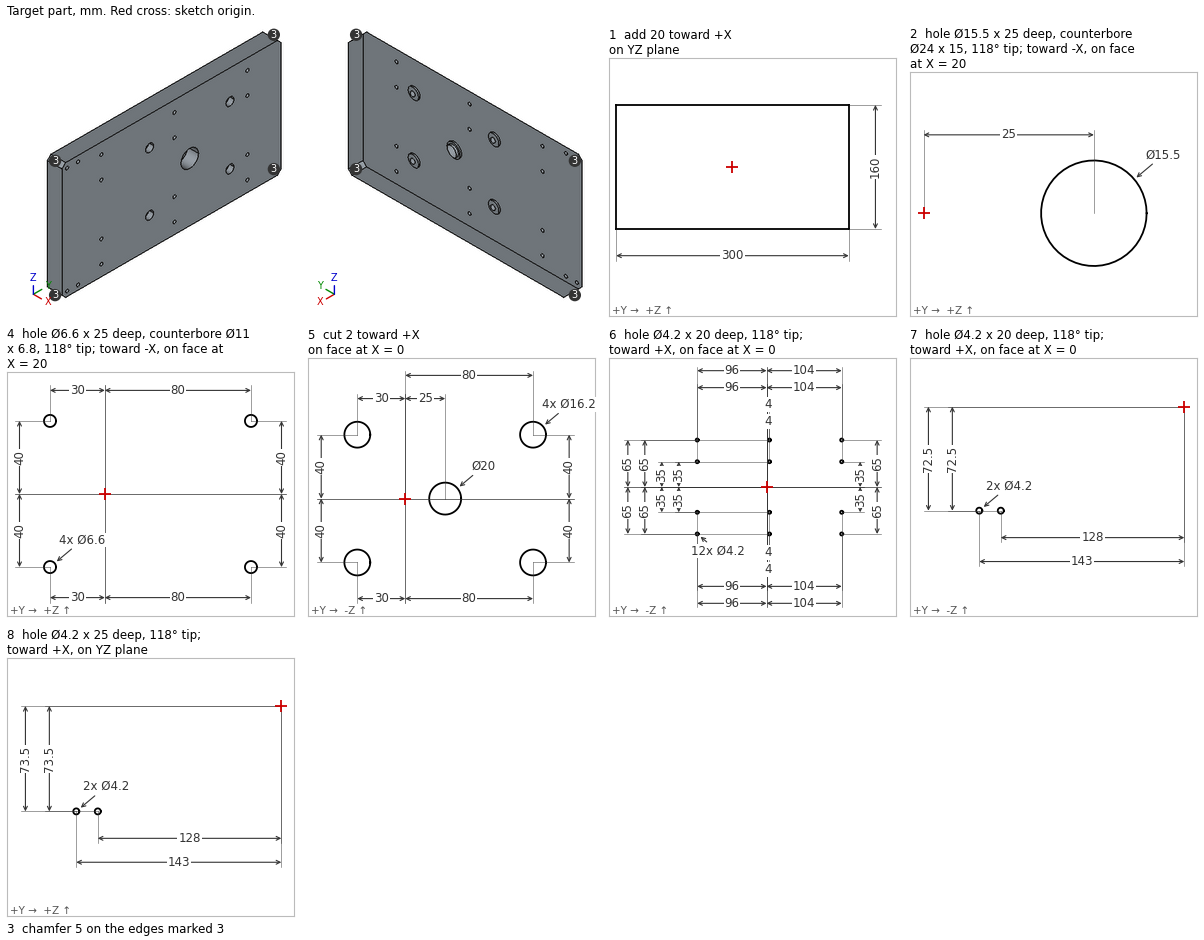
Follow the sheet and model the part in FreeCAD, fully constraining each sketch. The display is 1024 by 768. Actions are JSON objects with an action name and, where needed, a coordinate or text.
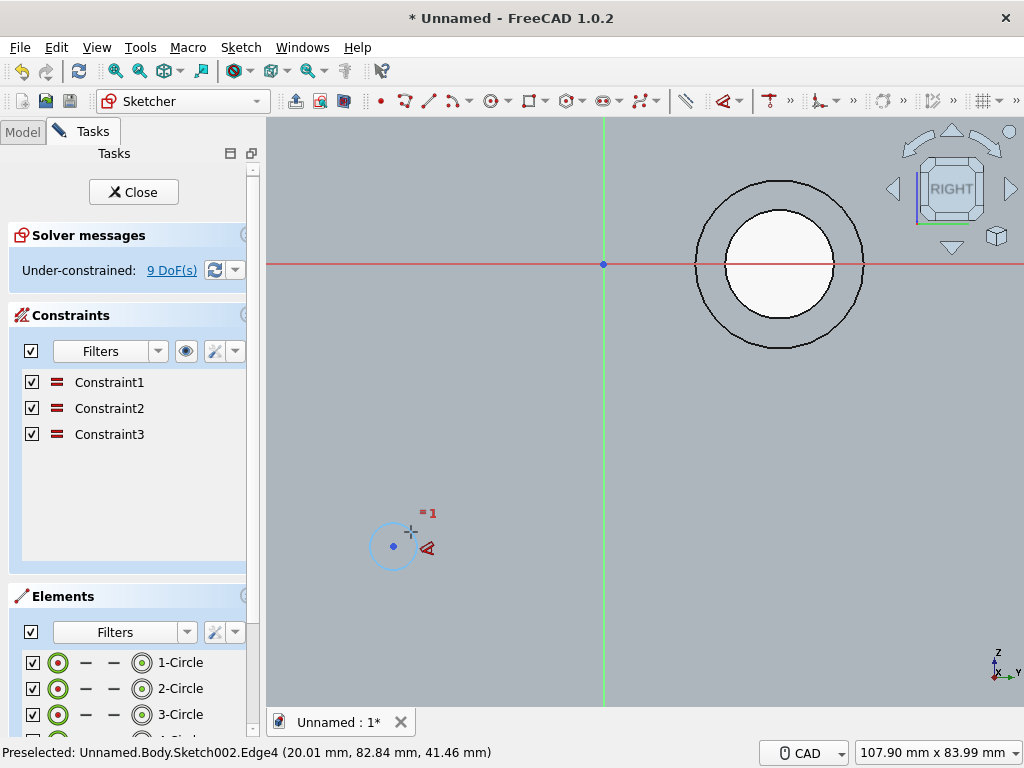
{"action": "left_click", "coordinate": [410, 530]}
{"action": "left_click", "coordinate": [433, 507]}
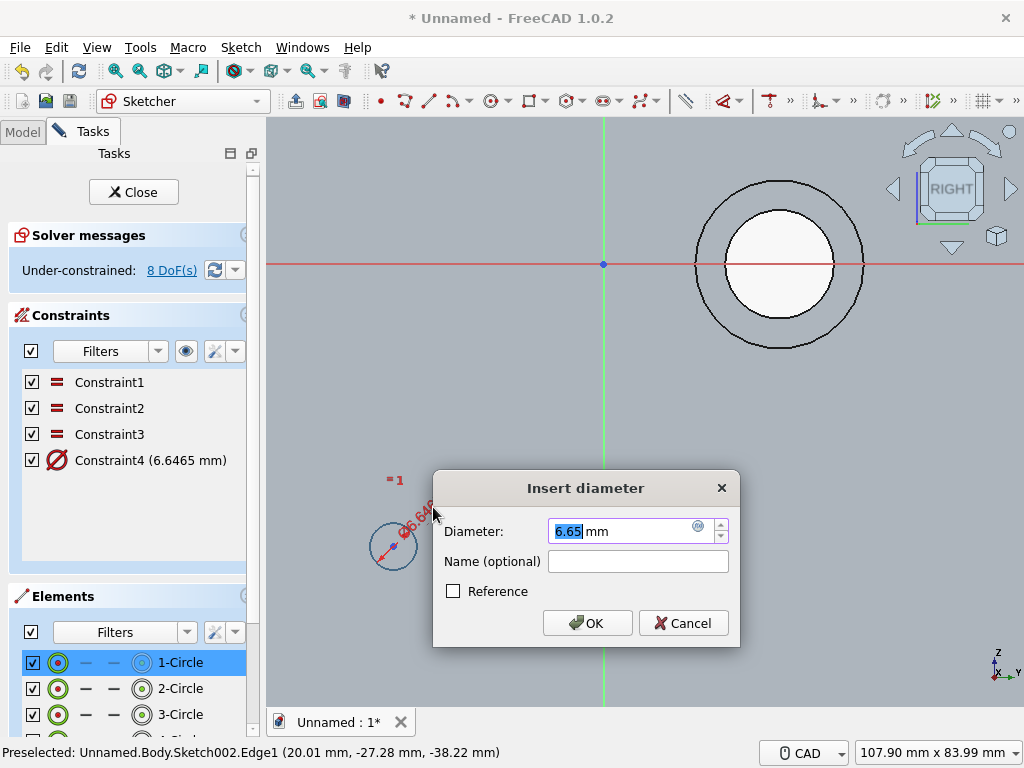
{"action": "type", "text": "6.6"}
{"action": "key", "text": "Return"}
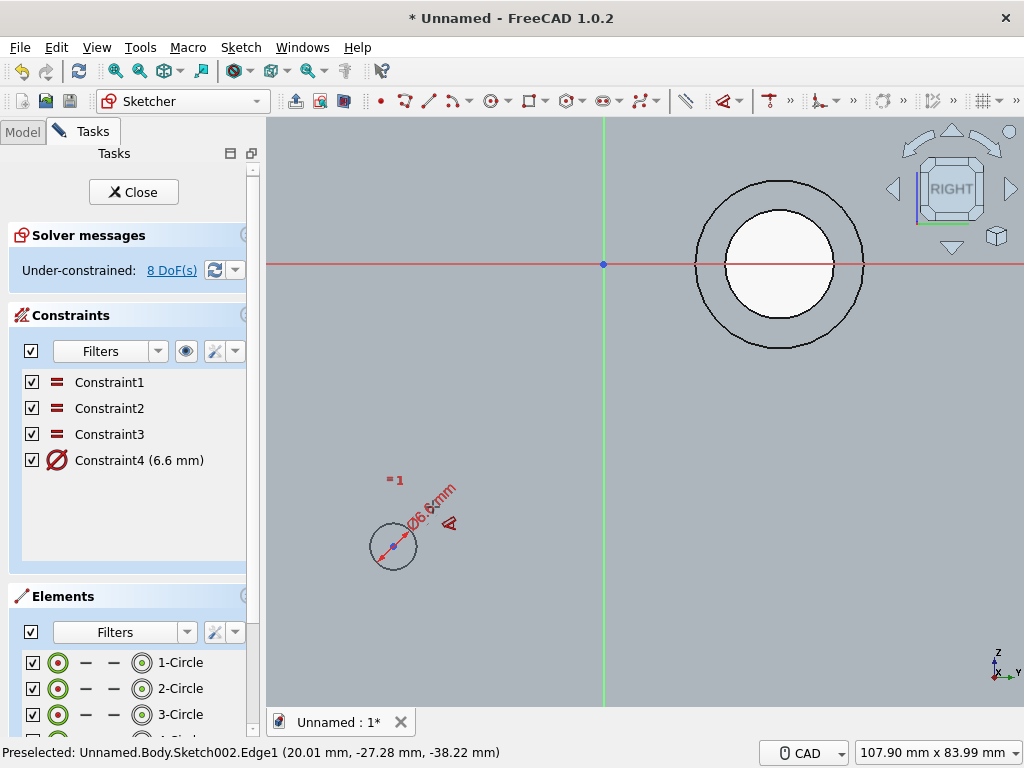
{"action": "left_click", "coordinate": [393, 547]}
{"action": "left_click", "coordinate": [499, 581]}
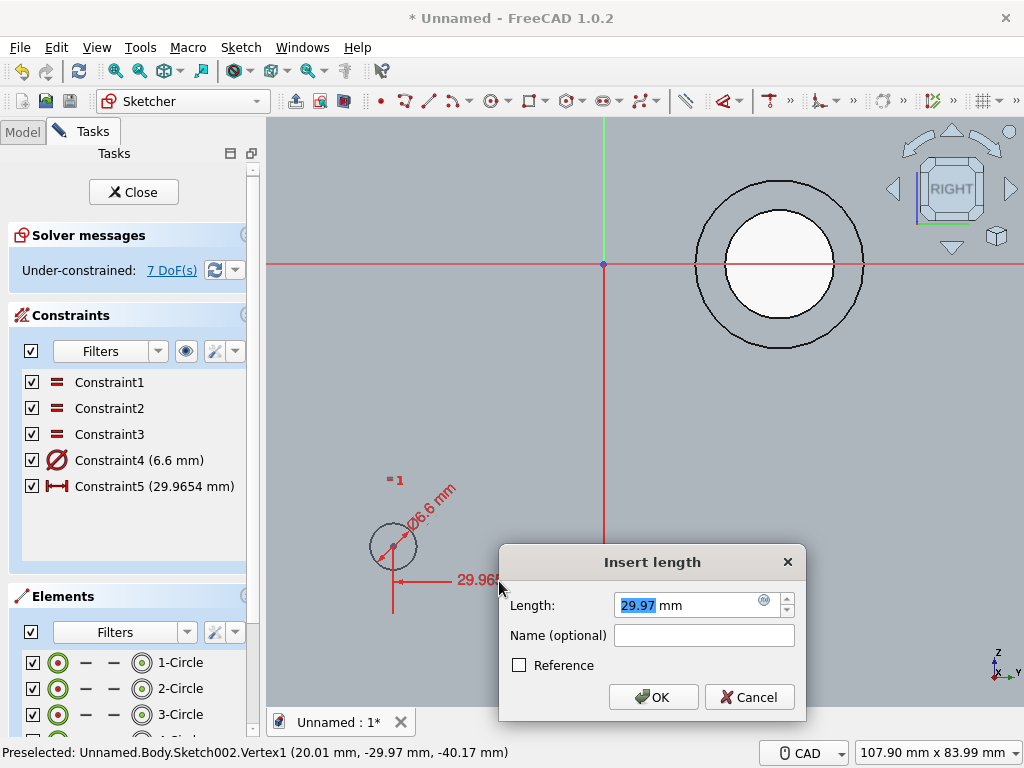
{"action": "type", "text": "30"}
{"action": "key", "text": "Return"}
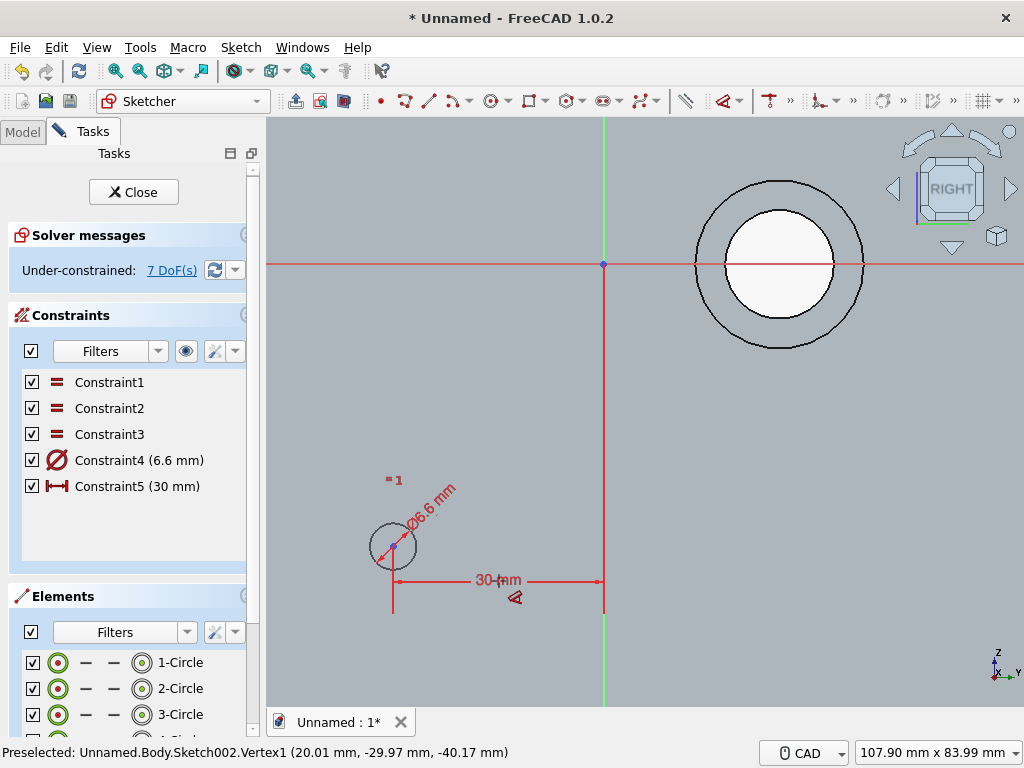
{"action": "left_click", "coordinate": [393, 547]}
{"action": "left_click", "coordinate": [359, 405]}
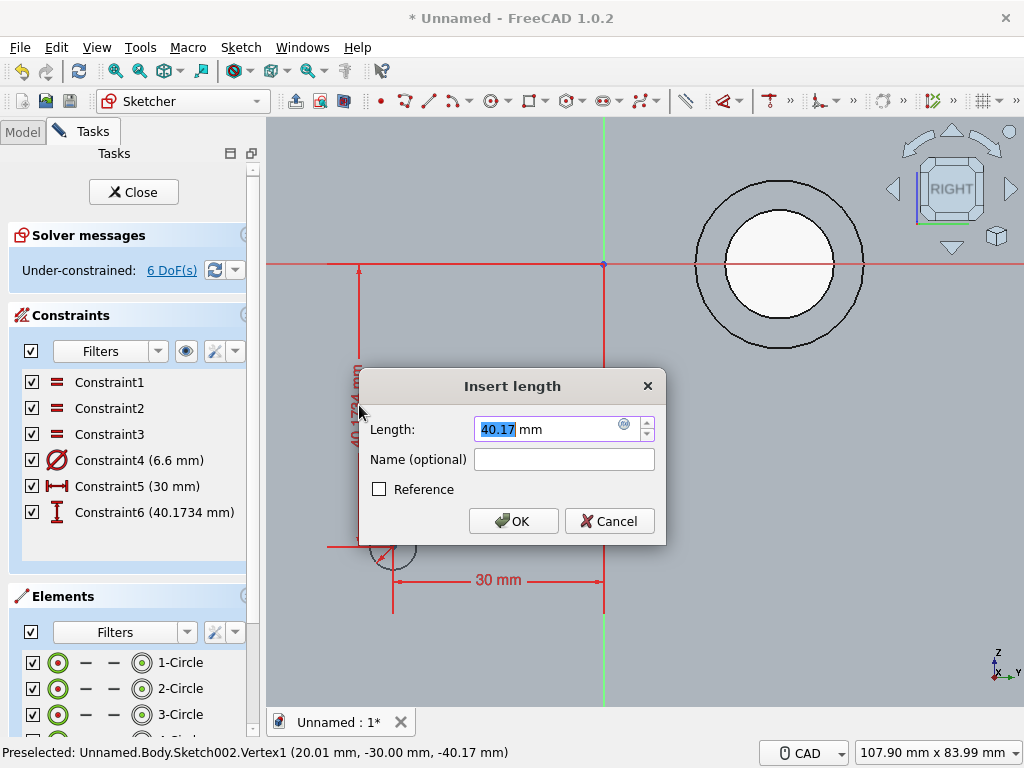
{"action": "type", "text": "40"}
{"action": "key", "text": "Return"}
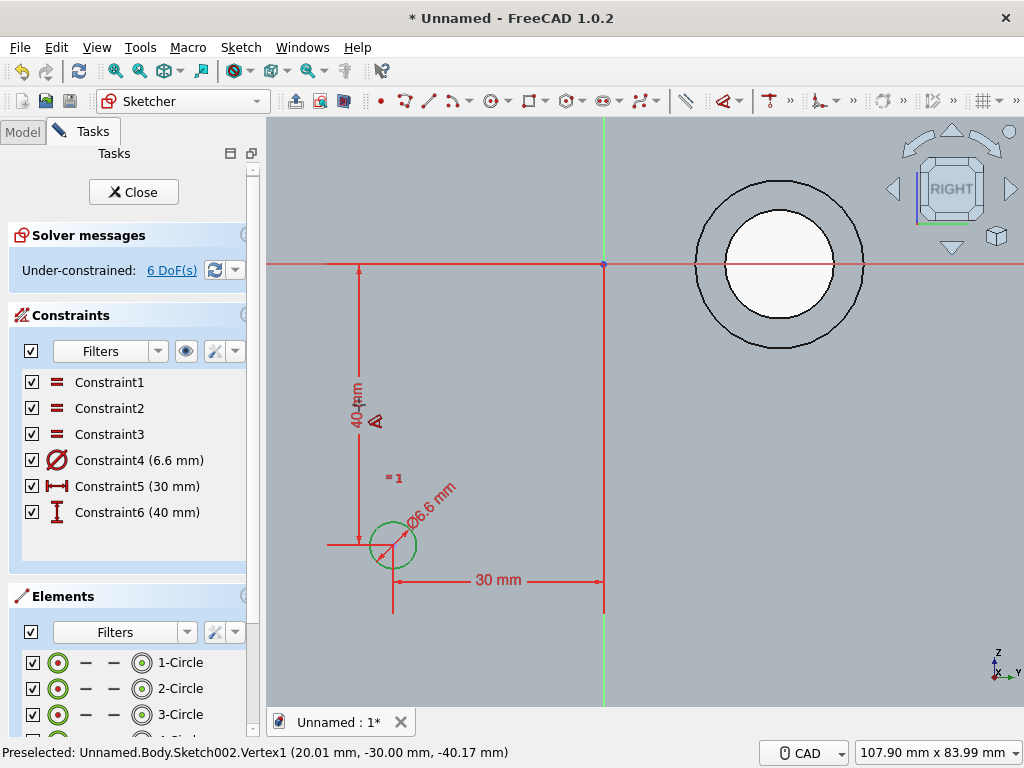
{"action": "scroll", "coordinate": [411, 532], "scroll_direction": "down", "scroll_amount": 4}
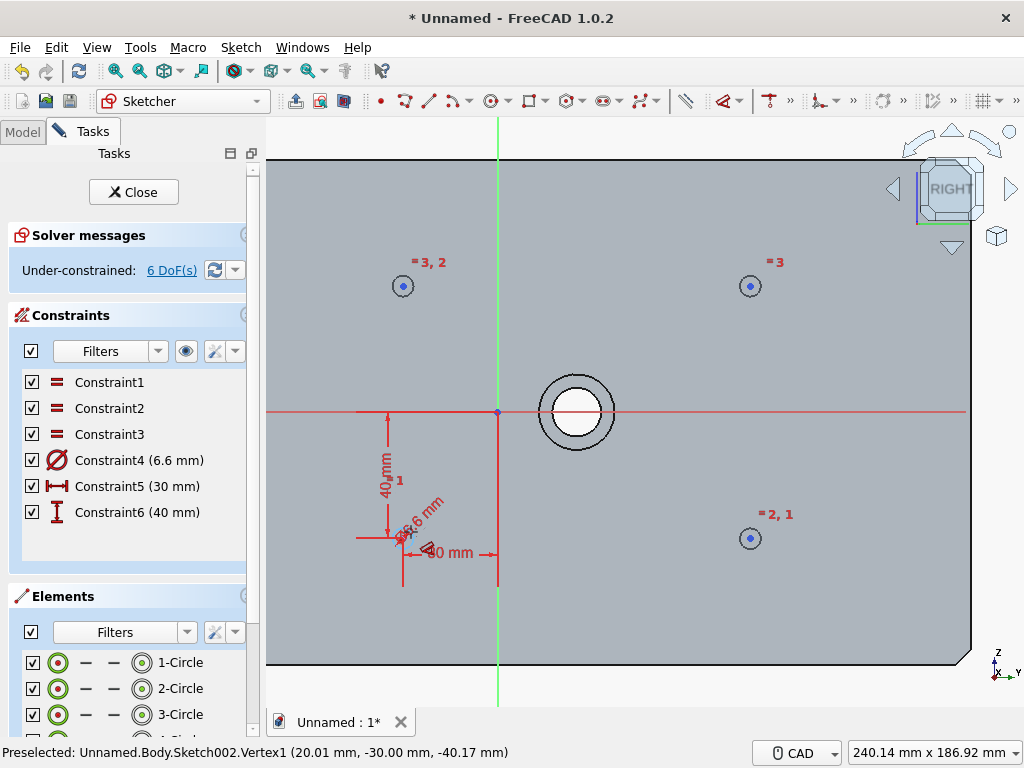
{"action": "left_click", "coordinate": [750, 539]}
{"action": "left_click", "coordinate": [624, 573]}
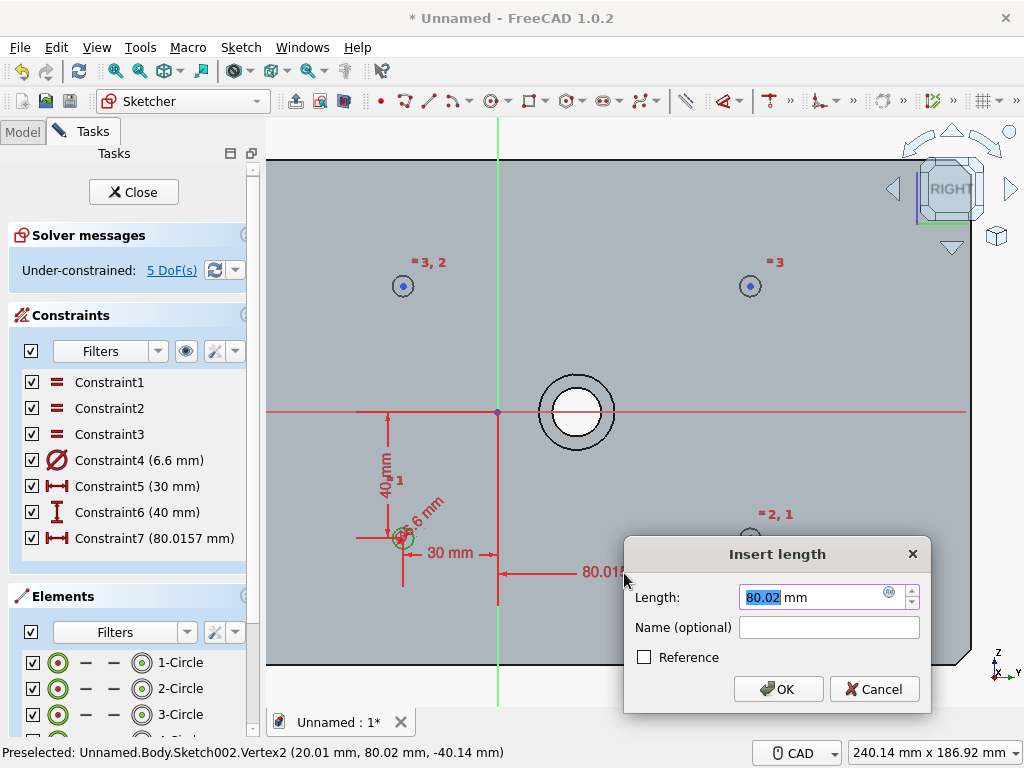
{"action": "type", "text": "80"}
{"action": "key", "text": "Return"}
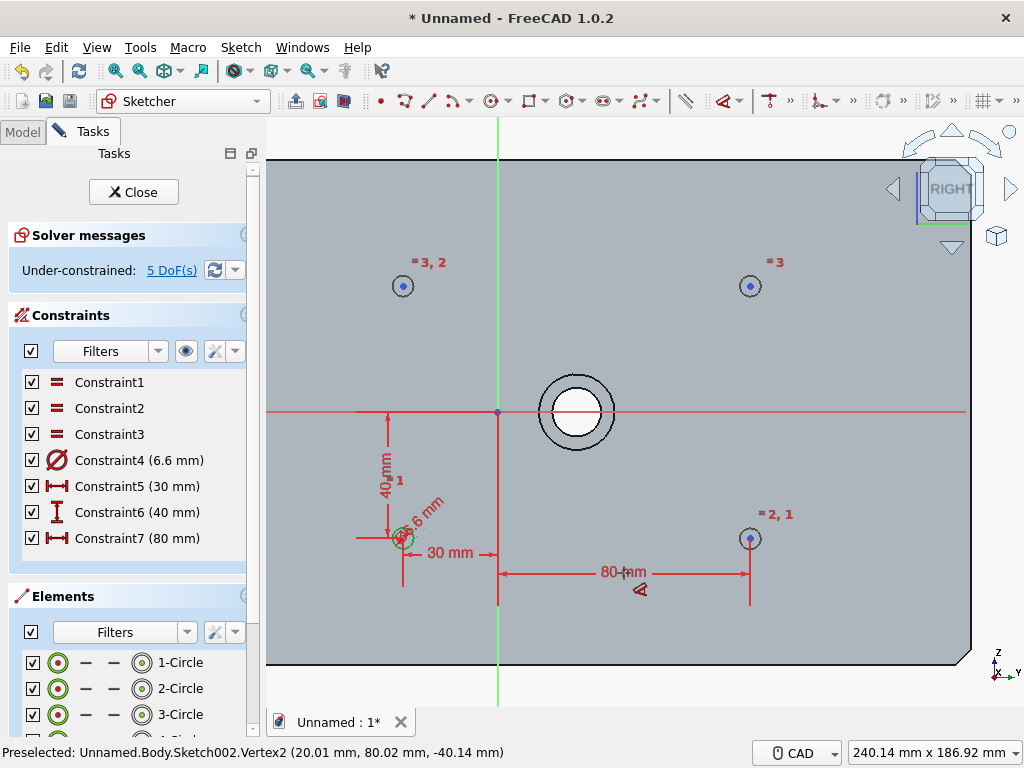
{"action": "left_click", "coordinate": [750, 539]}
{"action": "left_click", "coordinate": [784, 475]}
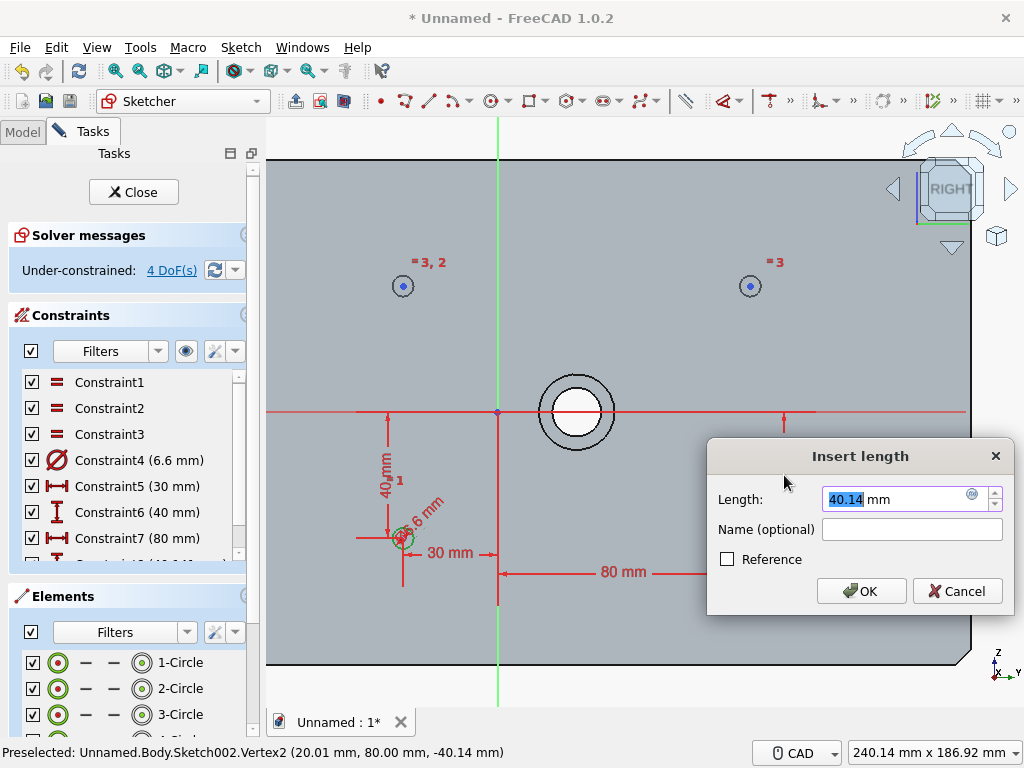
{"action": "type", "text": "40"}
{"action": "key", "text": "Return"}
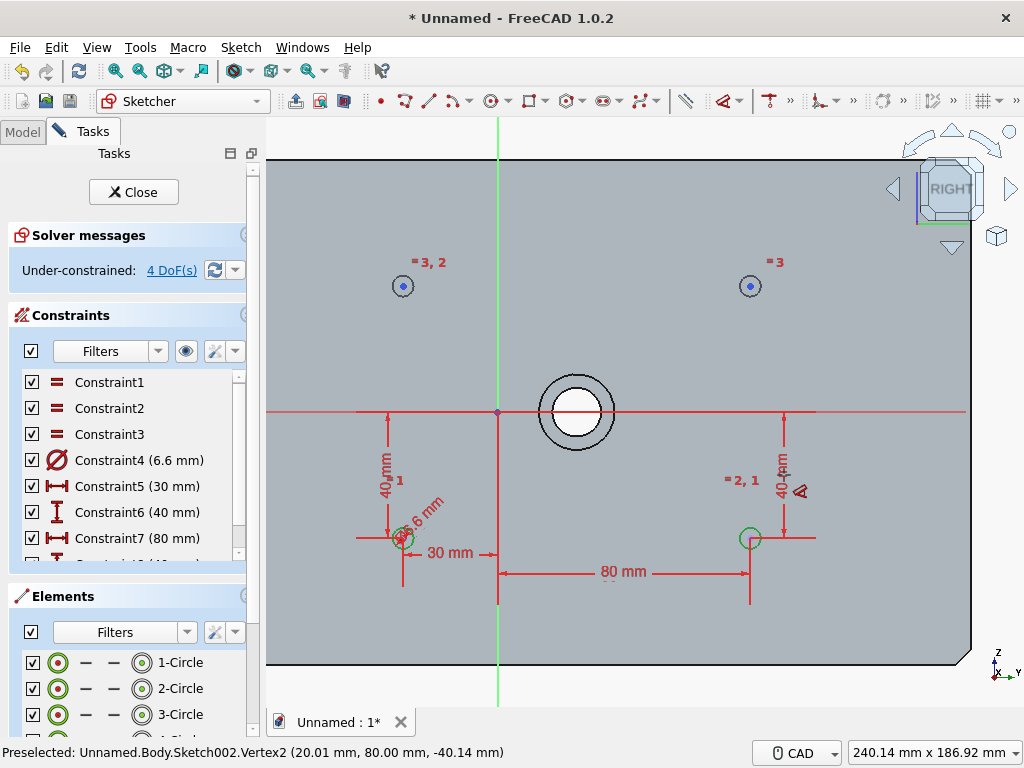
{"action": "left_click", "coordinate": [403, 286]}
{"action": "left_click", "coordinate": [450, 252]}